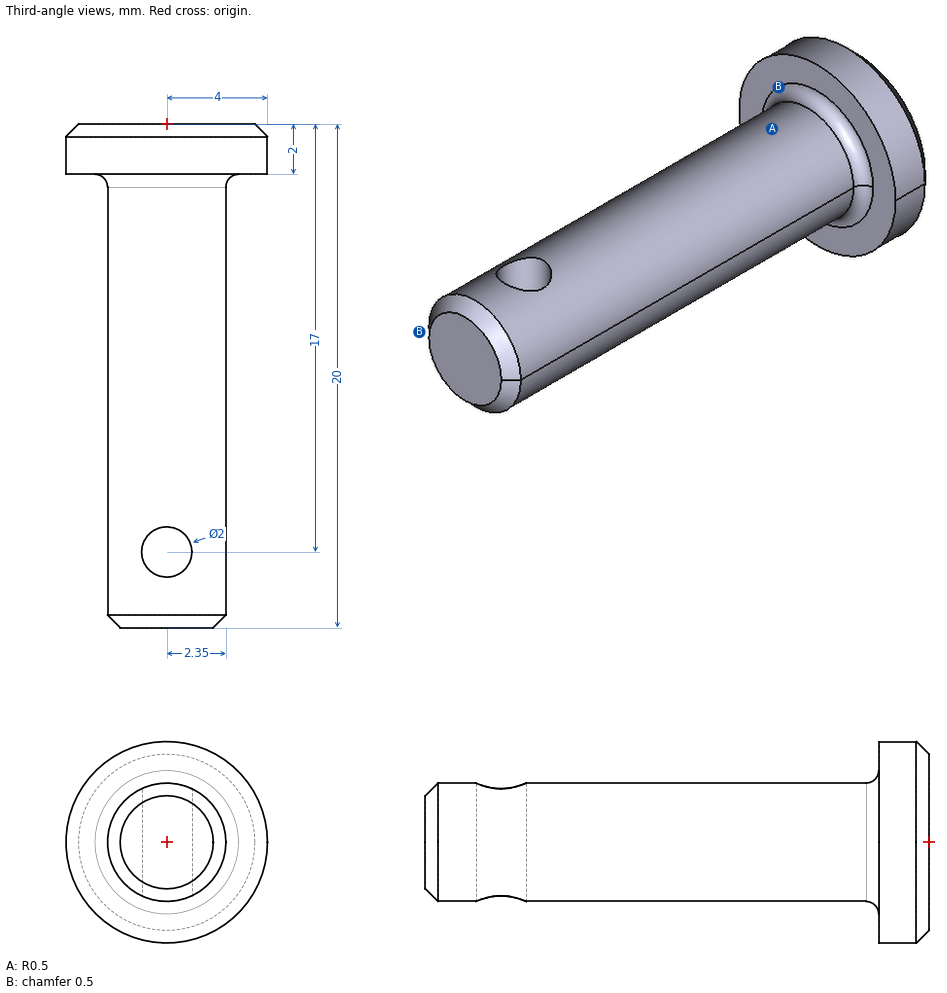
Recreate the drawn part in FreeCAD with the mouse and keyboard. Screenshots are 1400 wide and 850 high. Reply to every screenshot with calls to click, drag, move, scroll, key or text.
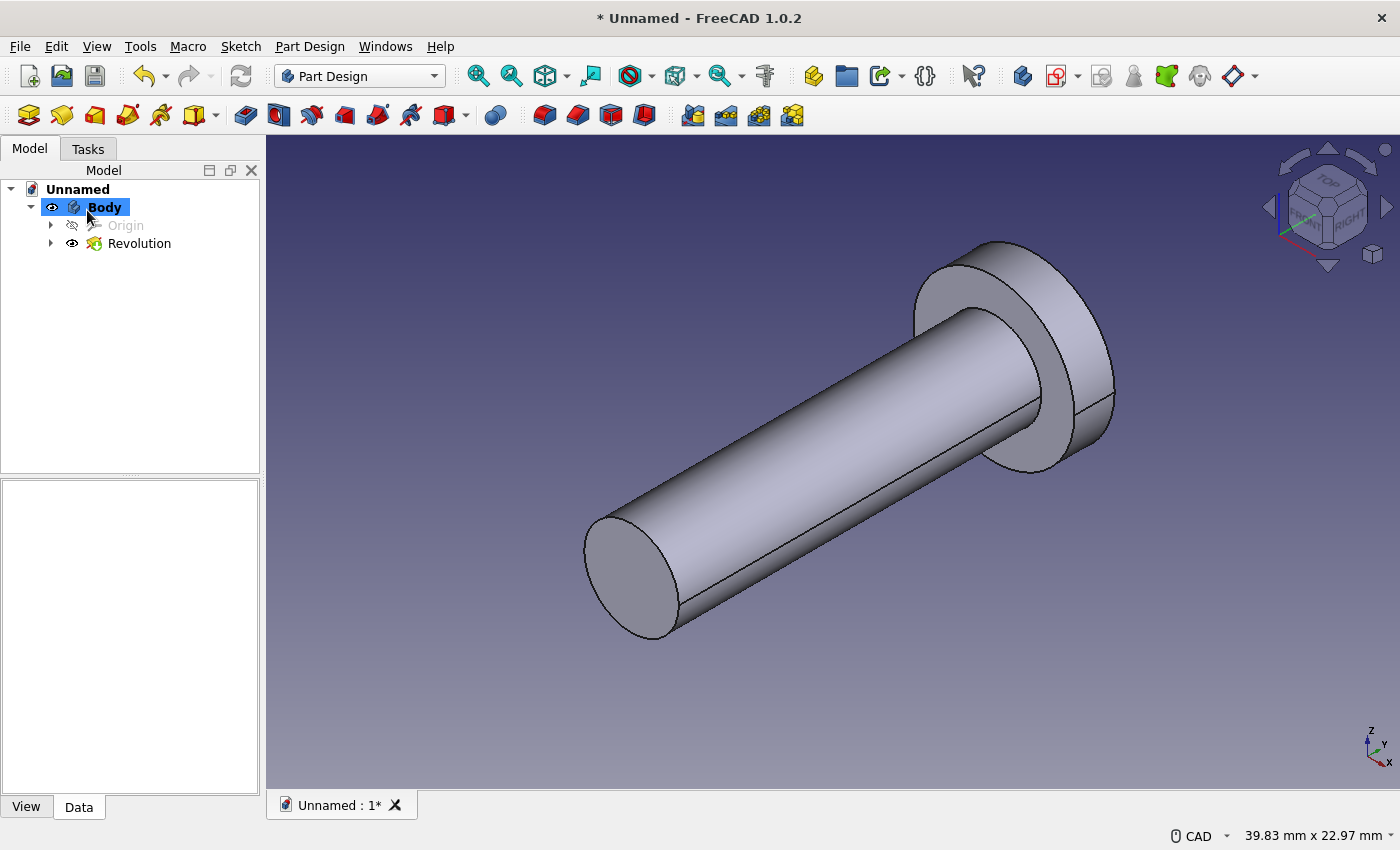
key(2)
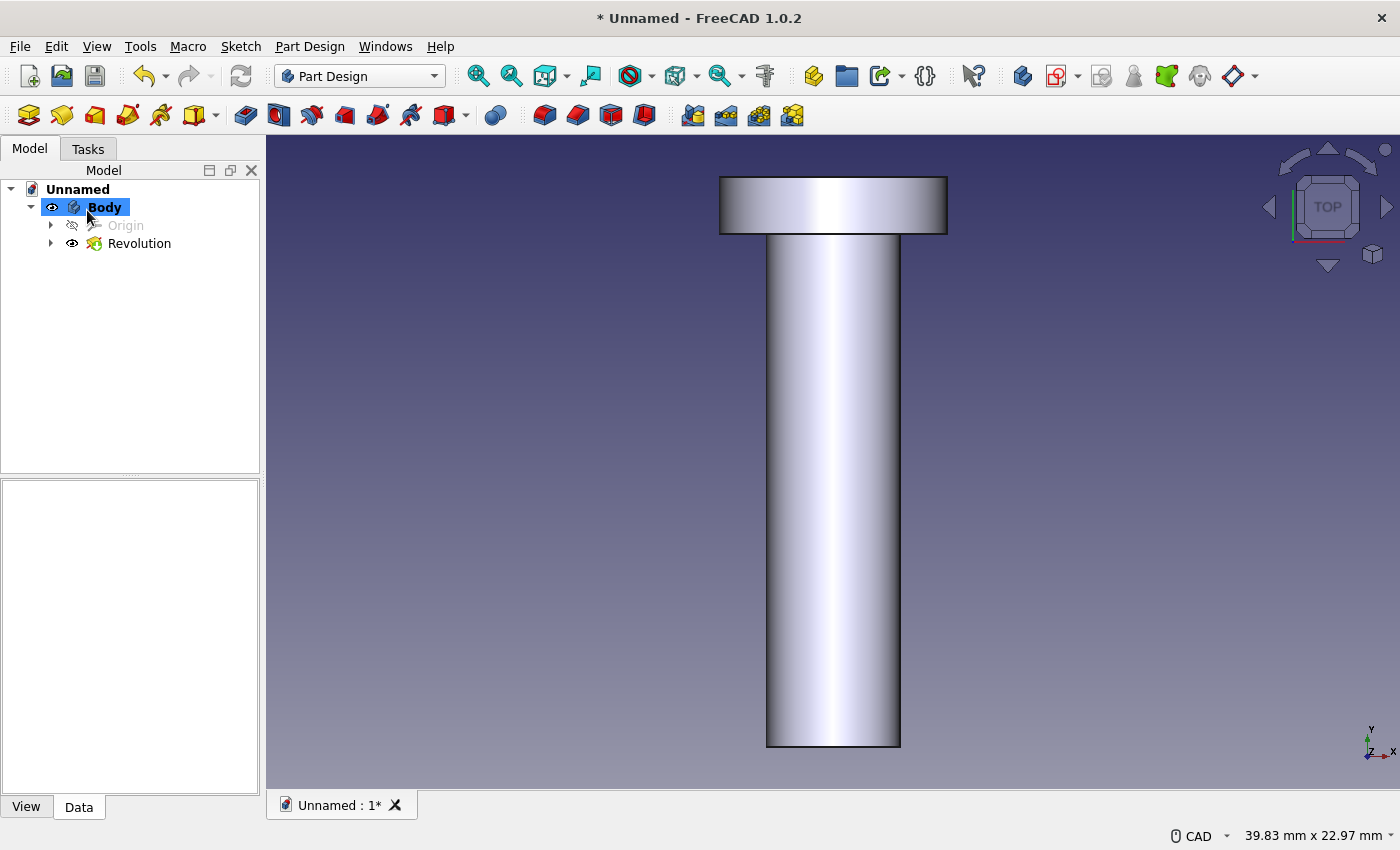
key(1)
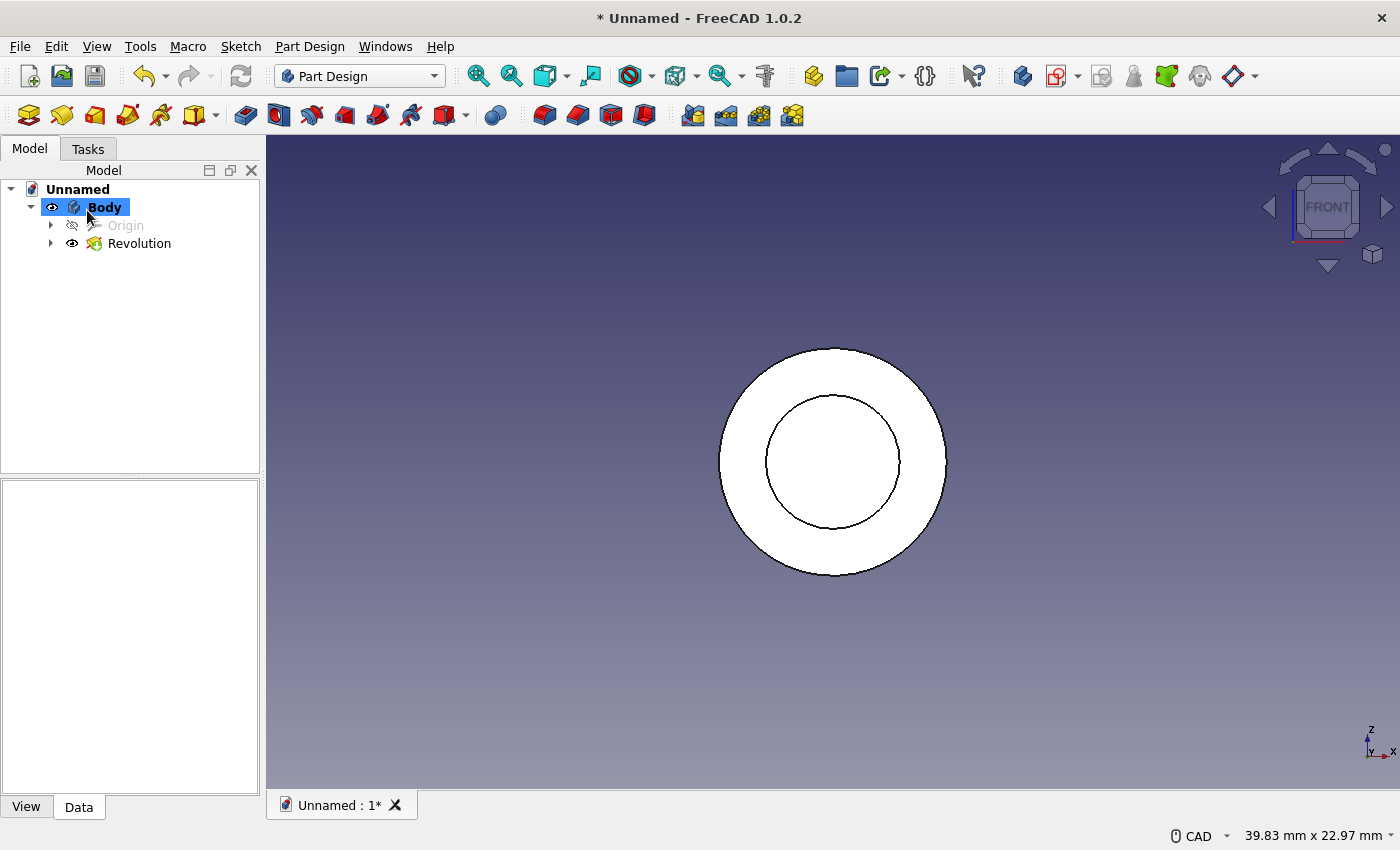
click(479, 76)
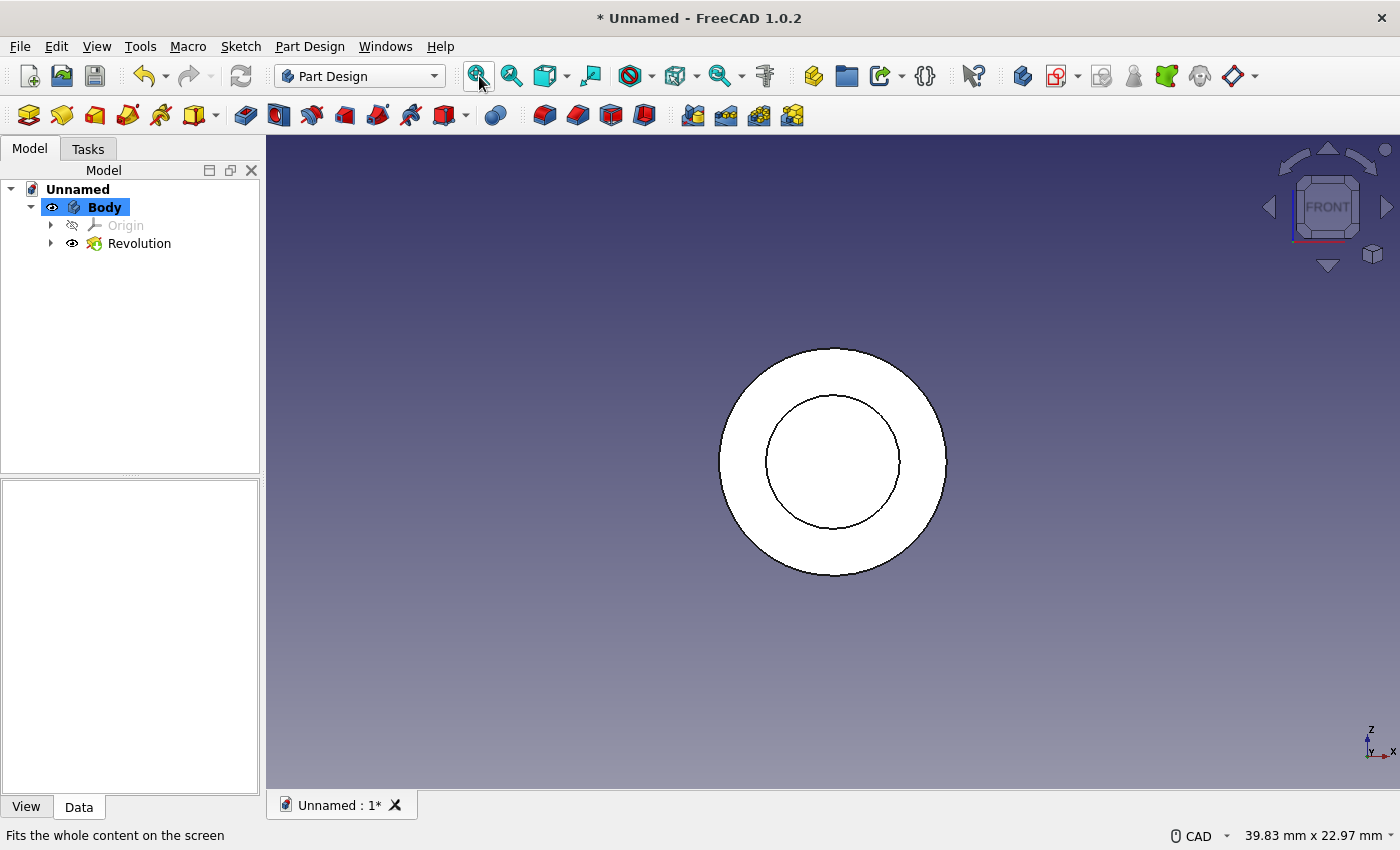
key(3)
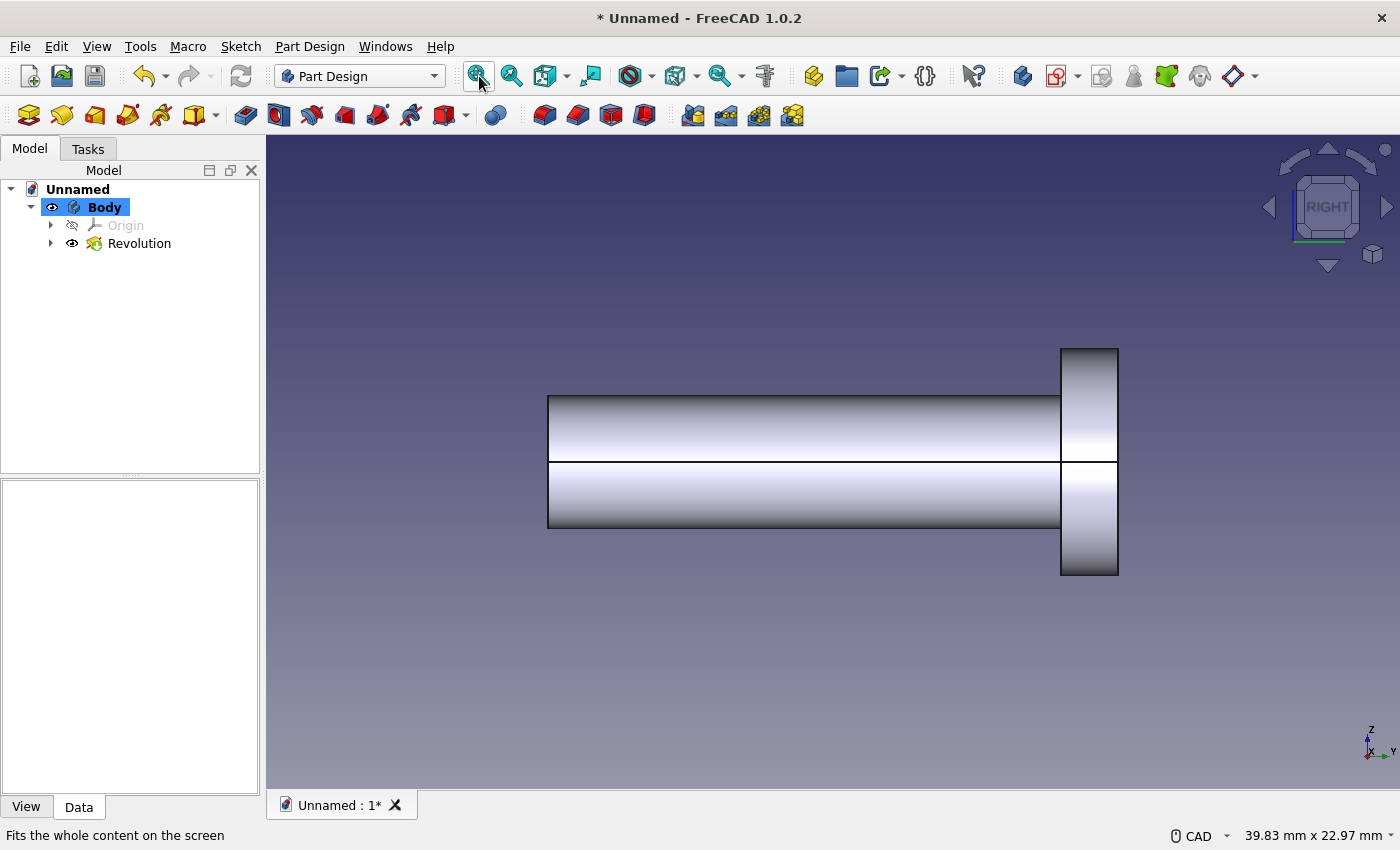
key(5)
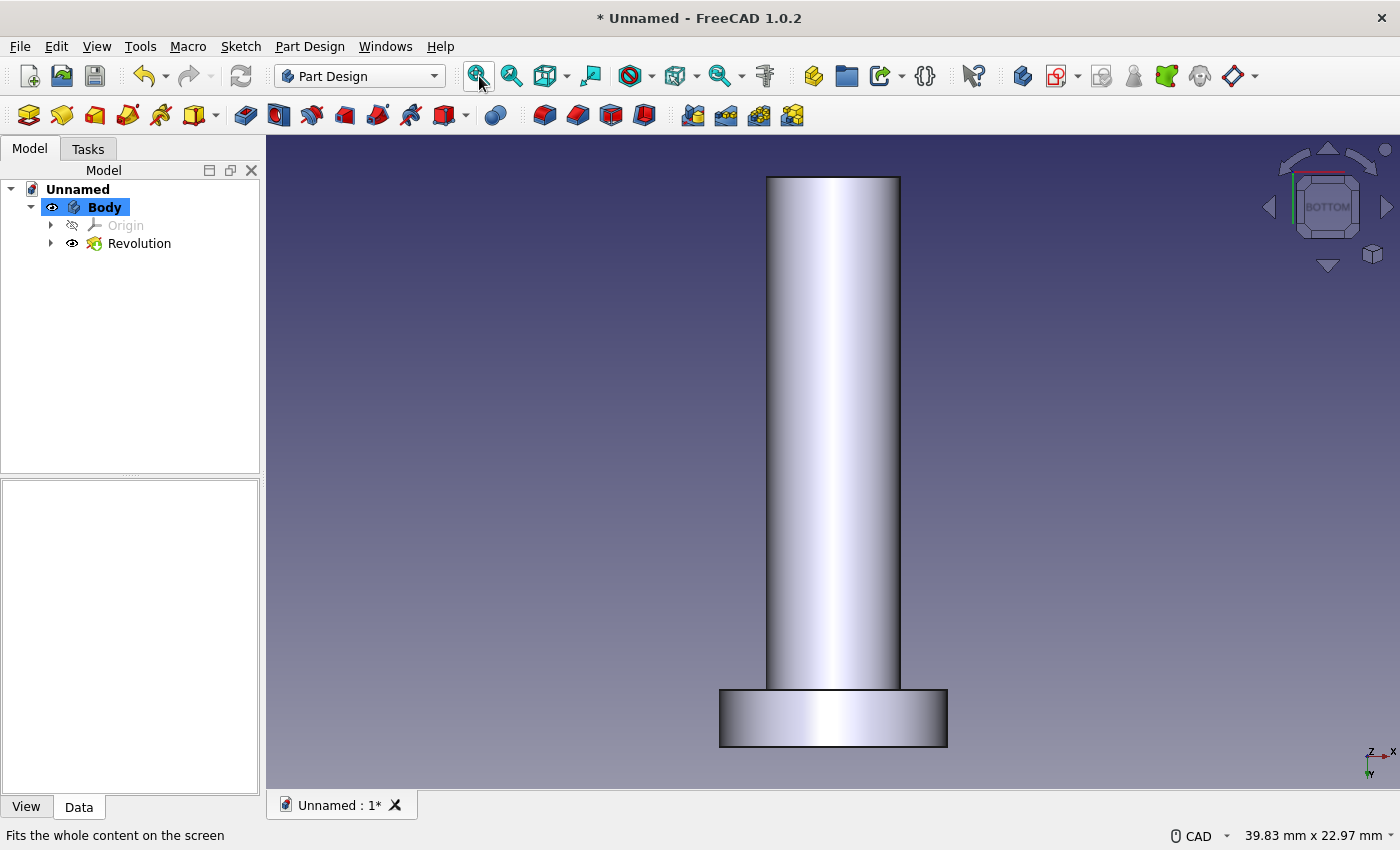
key(4)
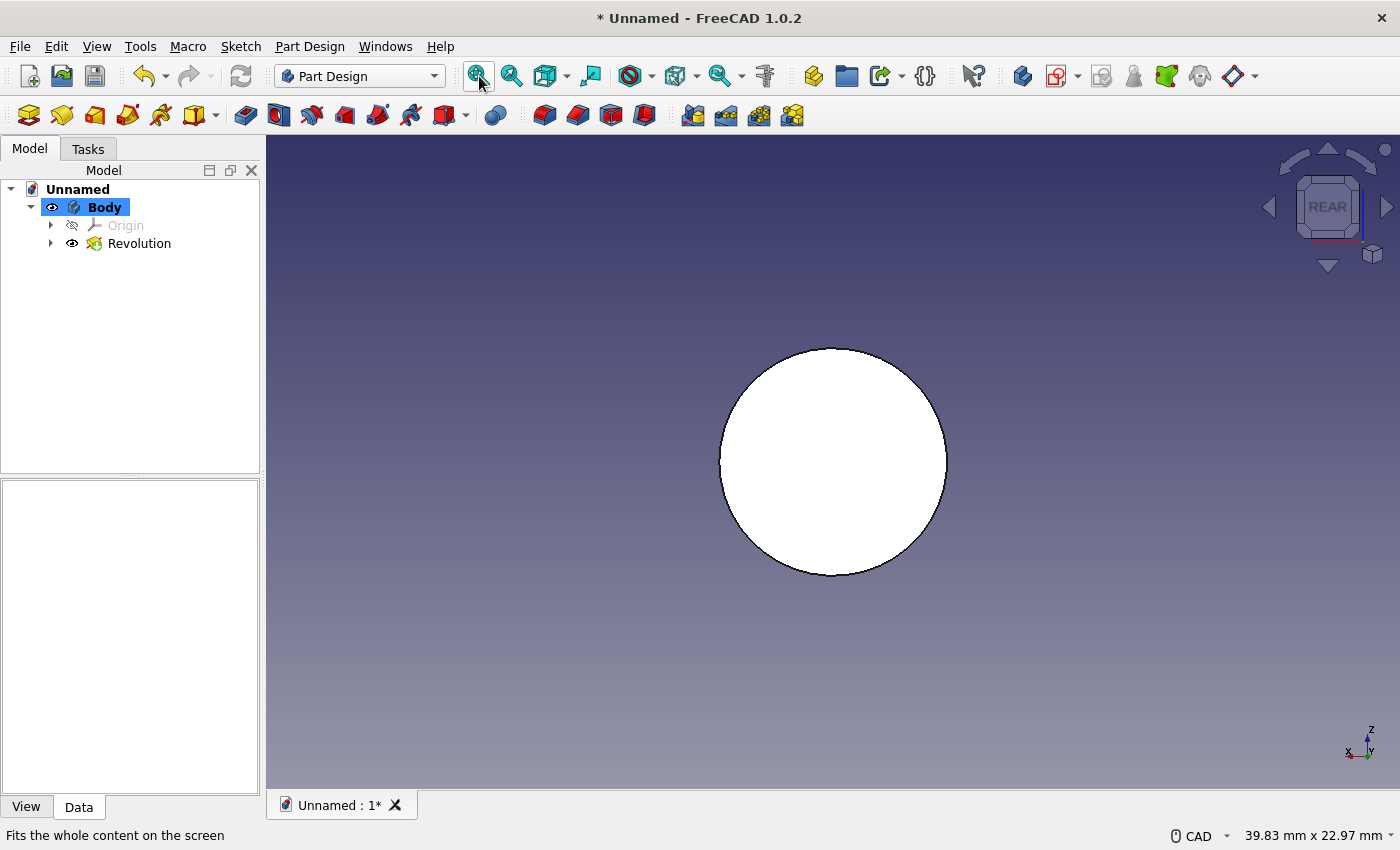
key(v)
key(f)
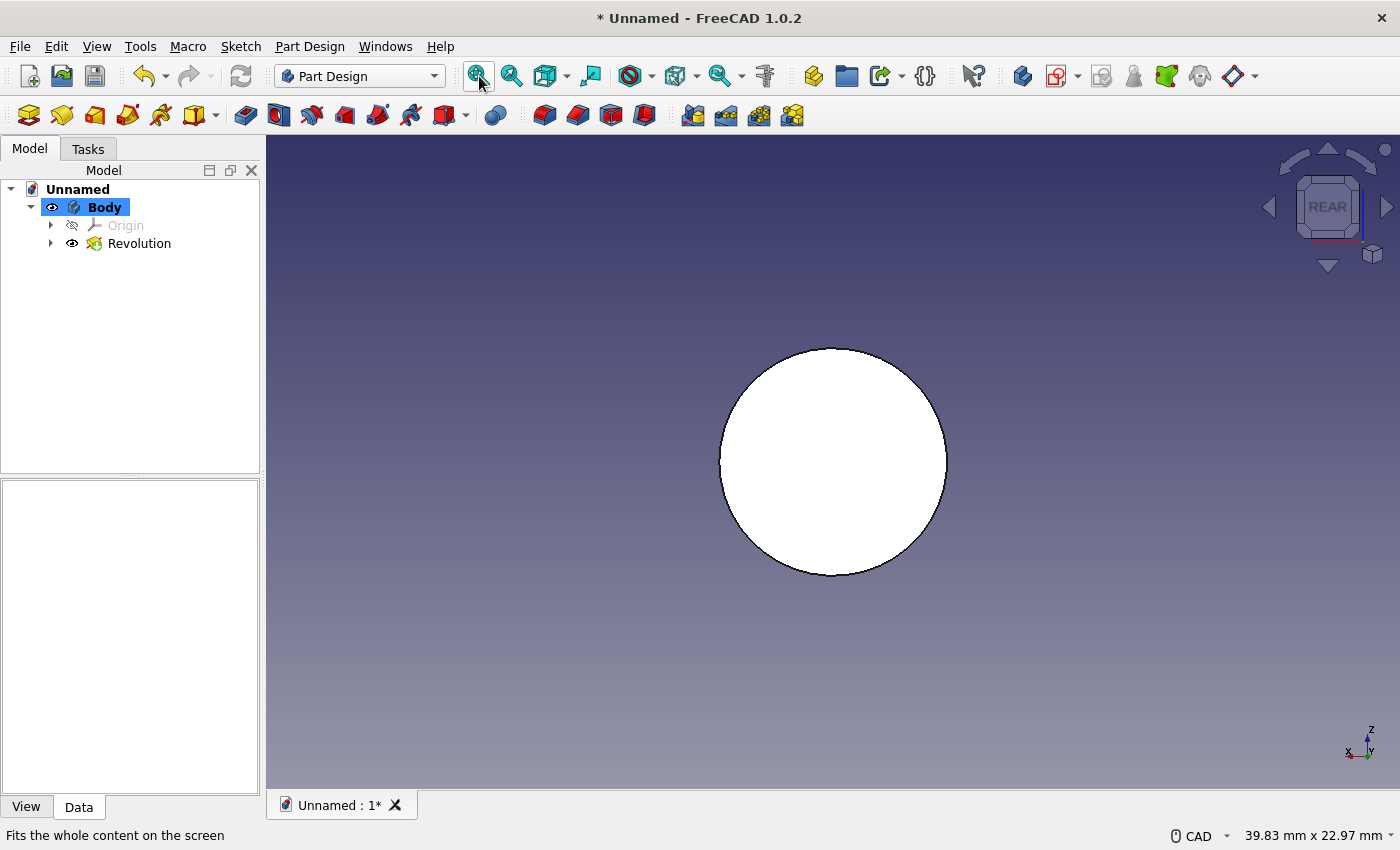
key(6)